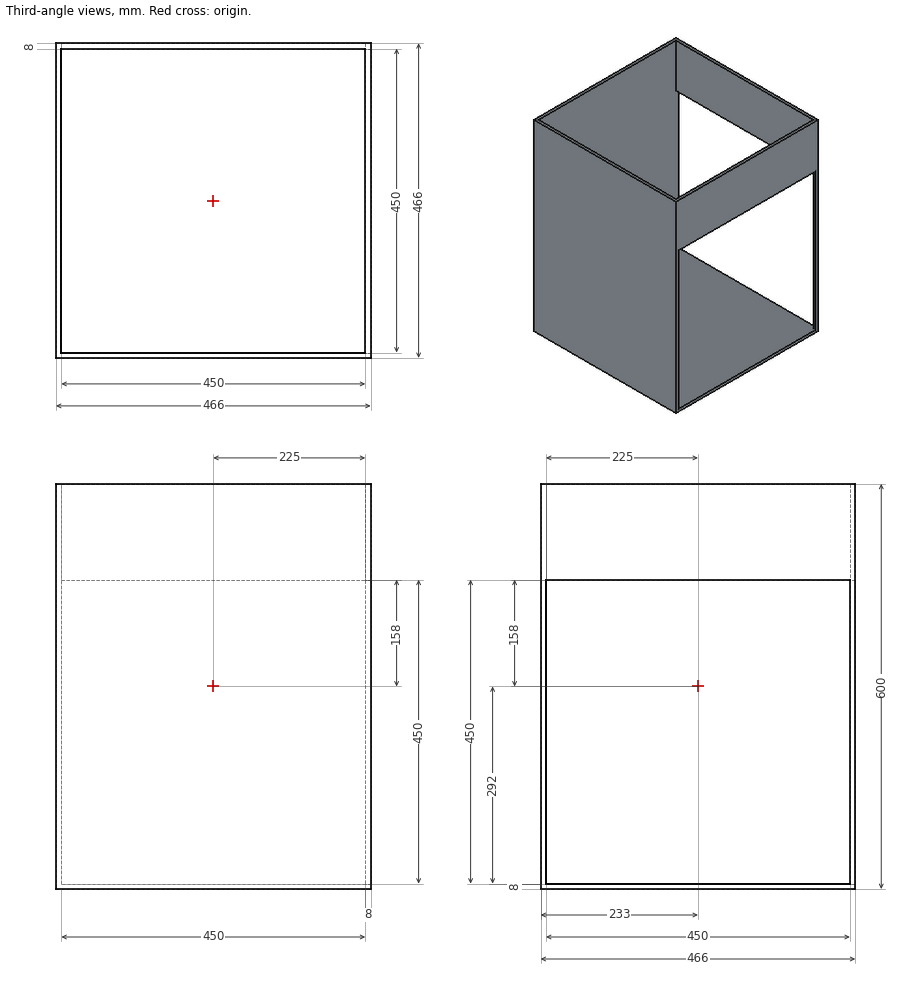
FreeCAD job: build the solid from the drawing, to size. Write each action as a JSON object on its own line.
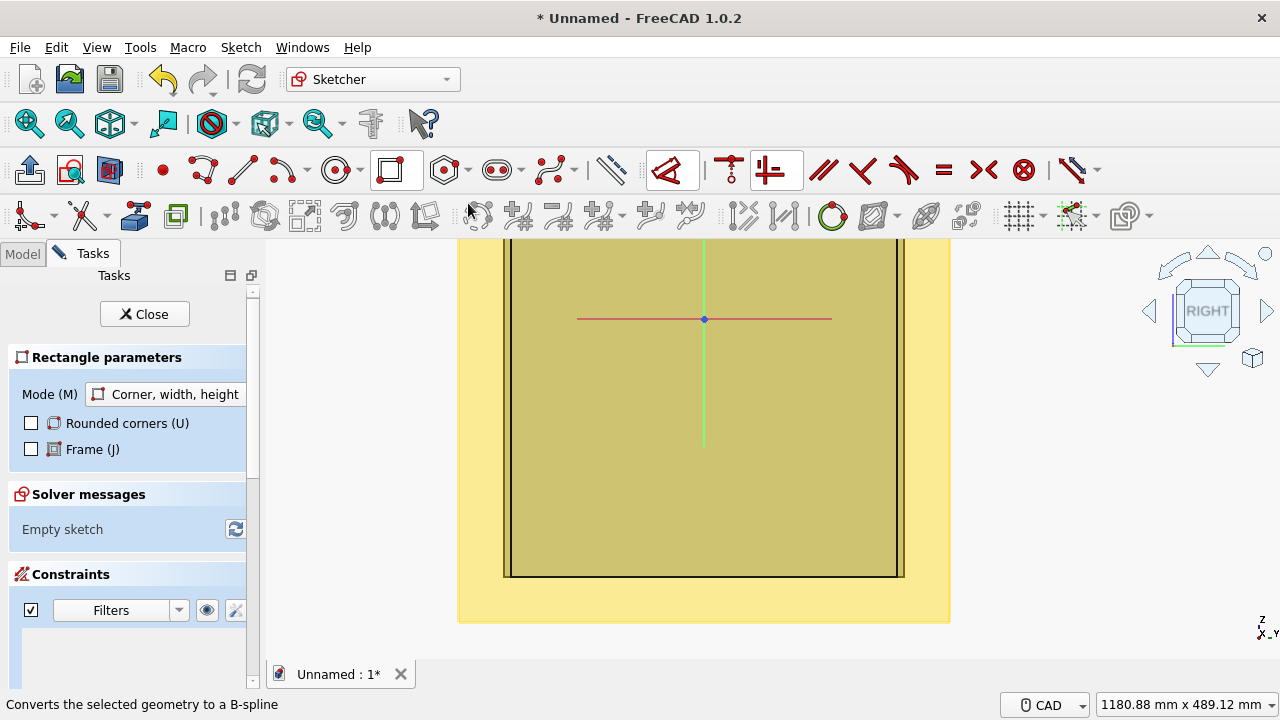
{"action": "scroll", "coordinate": [504, 570], "scroll_direction": "up", "scroll_amount": 5}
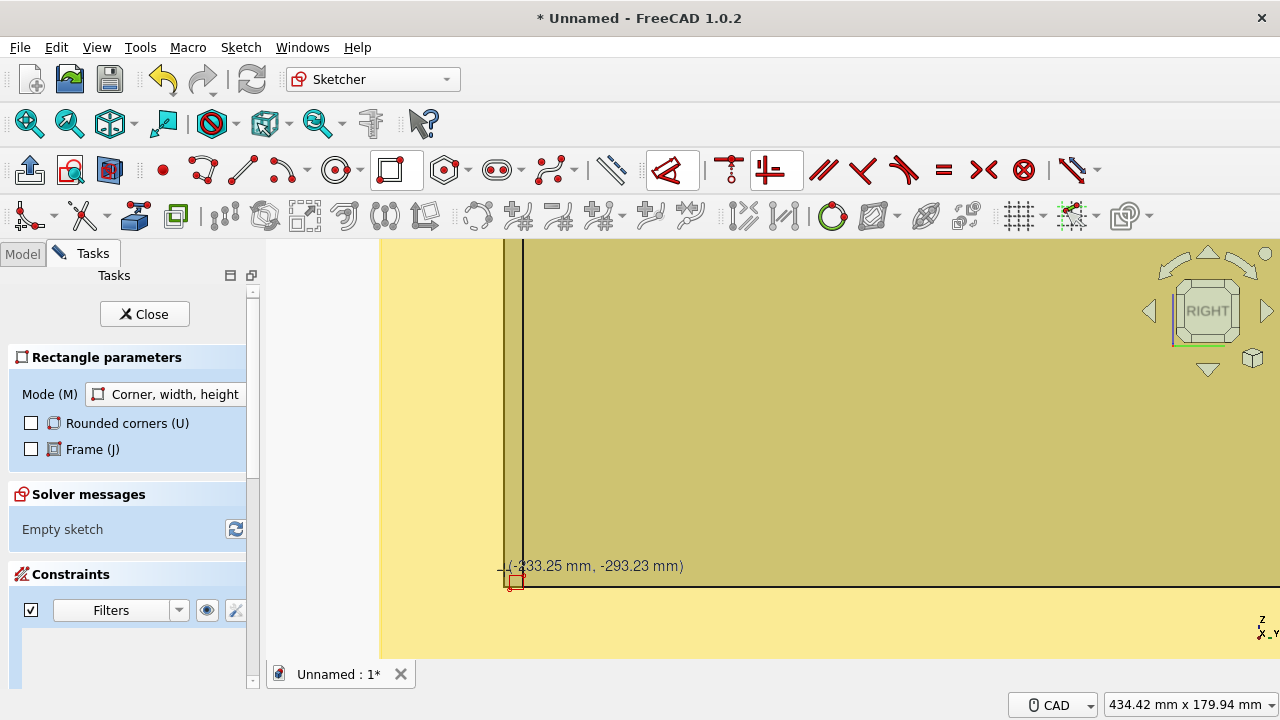
{"action": "left_click", "coordinate": [504, 568]}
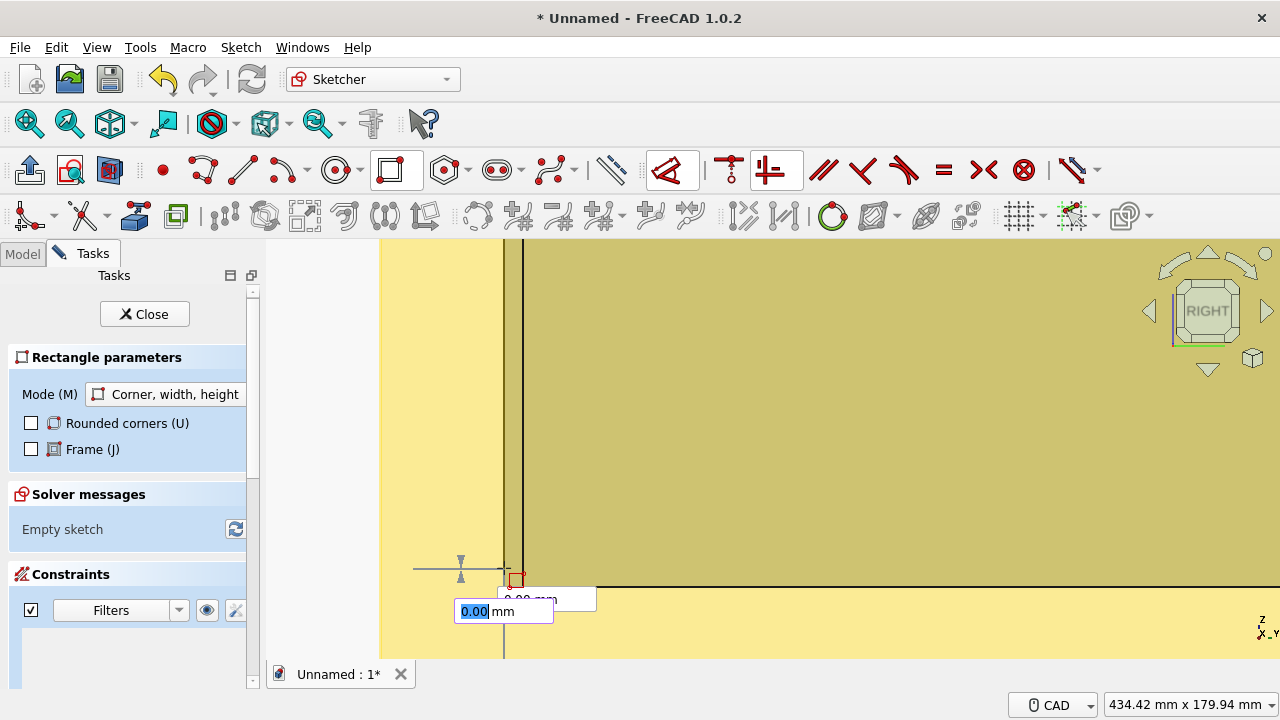
{"action": "scroll", "coordinate": [505, 572], "scroll_direction": "down", "scroll_amount": 5}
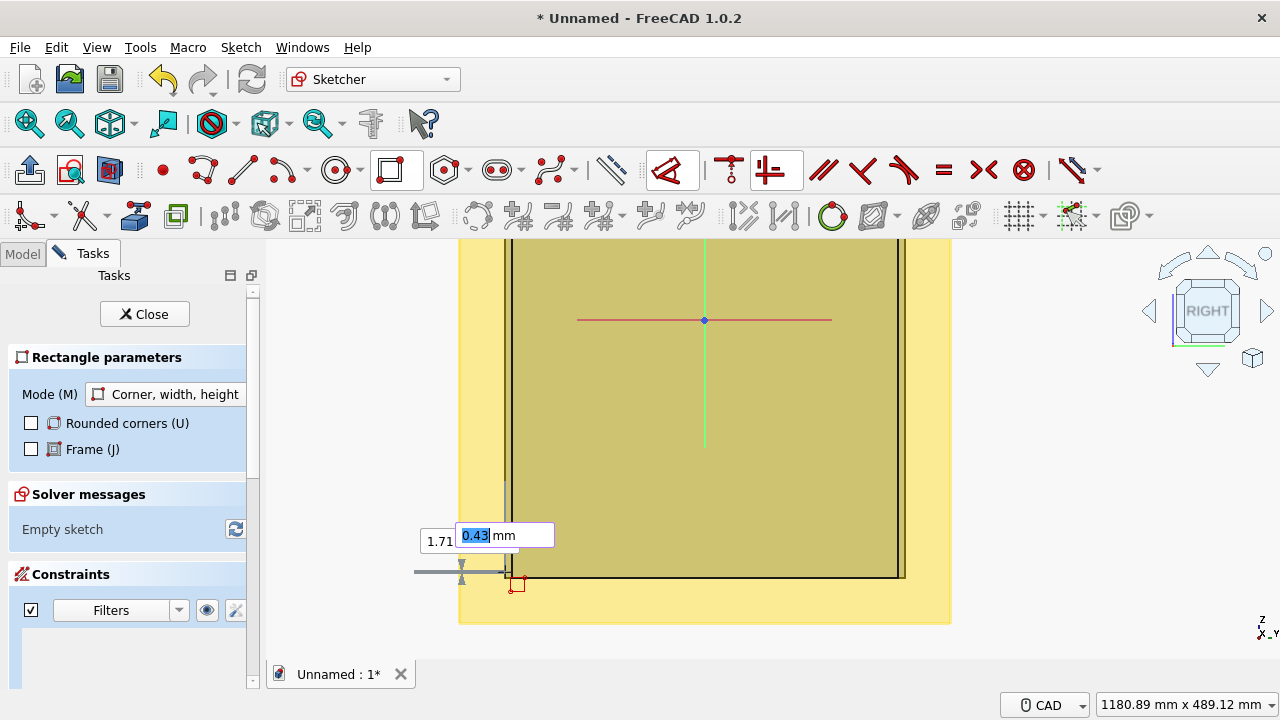
{"action": "left_click", "coordinate": [905, 578]}
{"action": "key", "text": "Escape"}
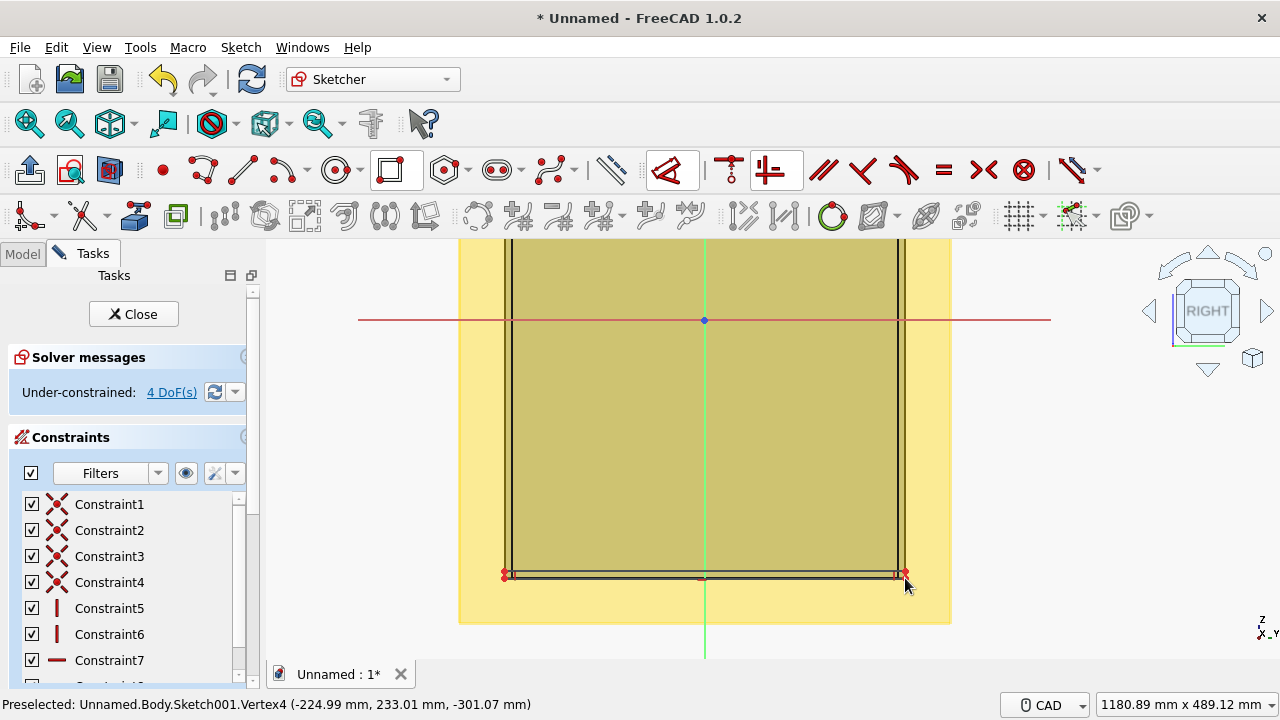
{"action": "scroll", "coordinate": [505, 575], "scroll_direction": "up", "scroll_amount": 9}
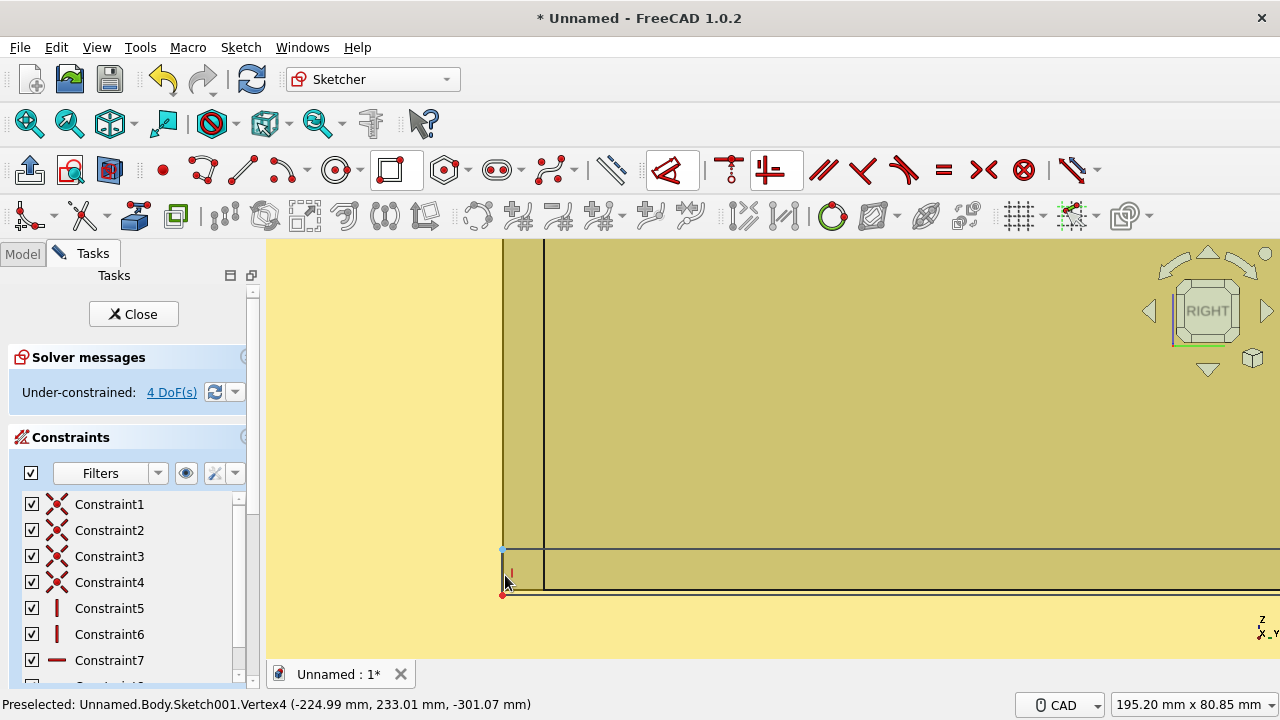
{"action": "left_click", "coordinate": [502, 572]}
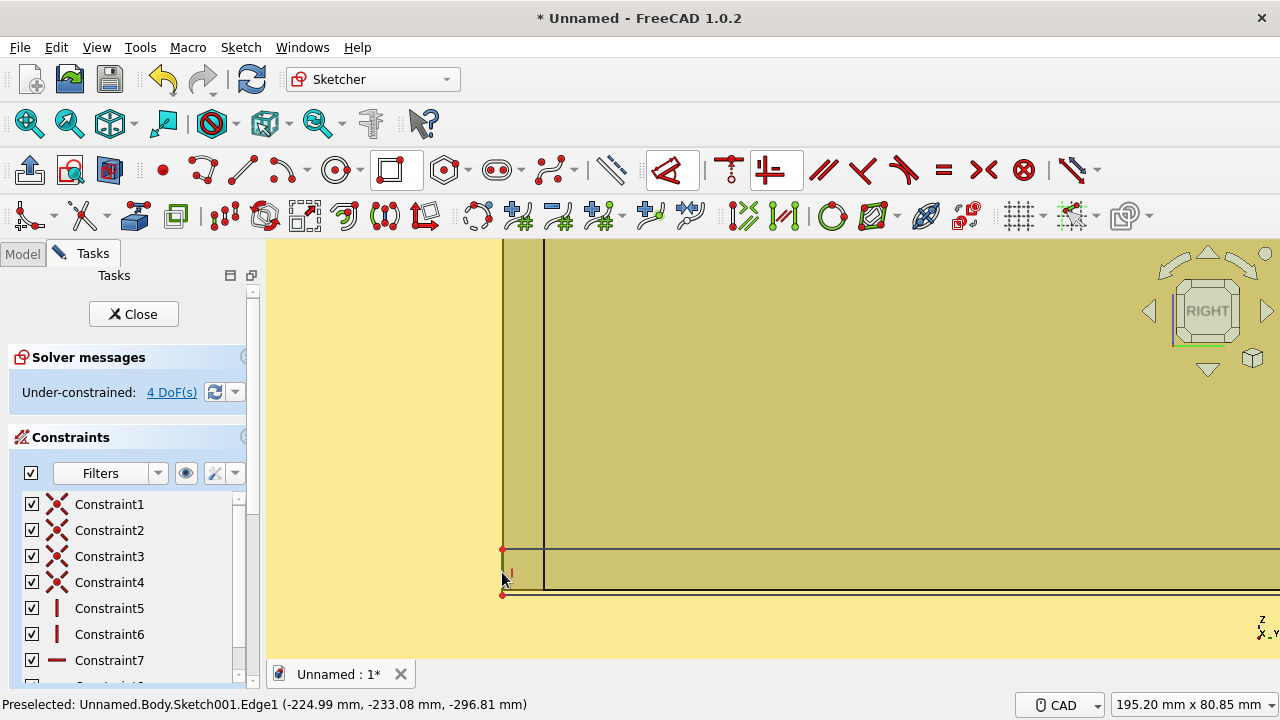
{"action": "key", "text": "i"}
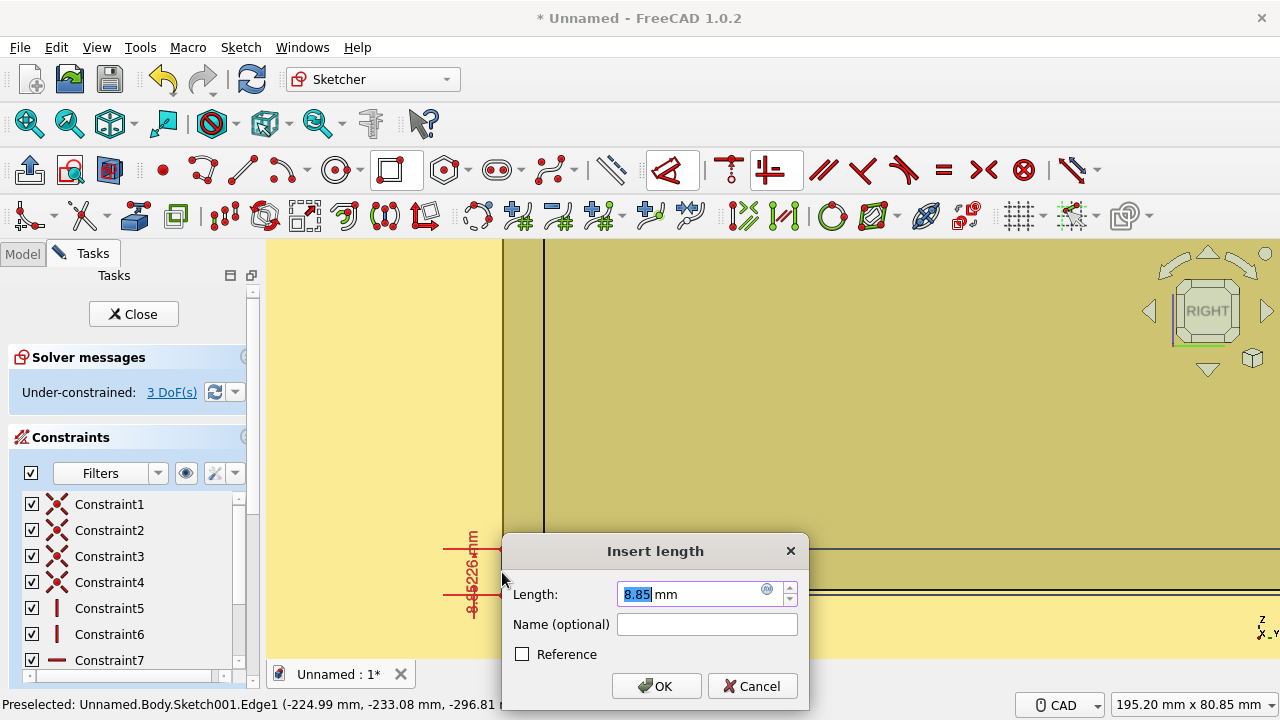
{"action": "type", "text": "8"}
{"action": "key", "text": "Return"}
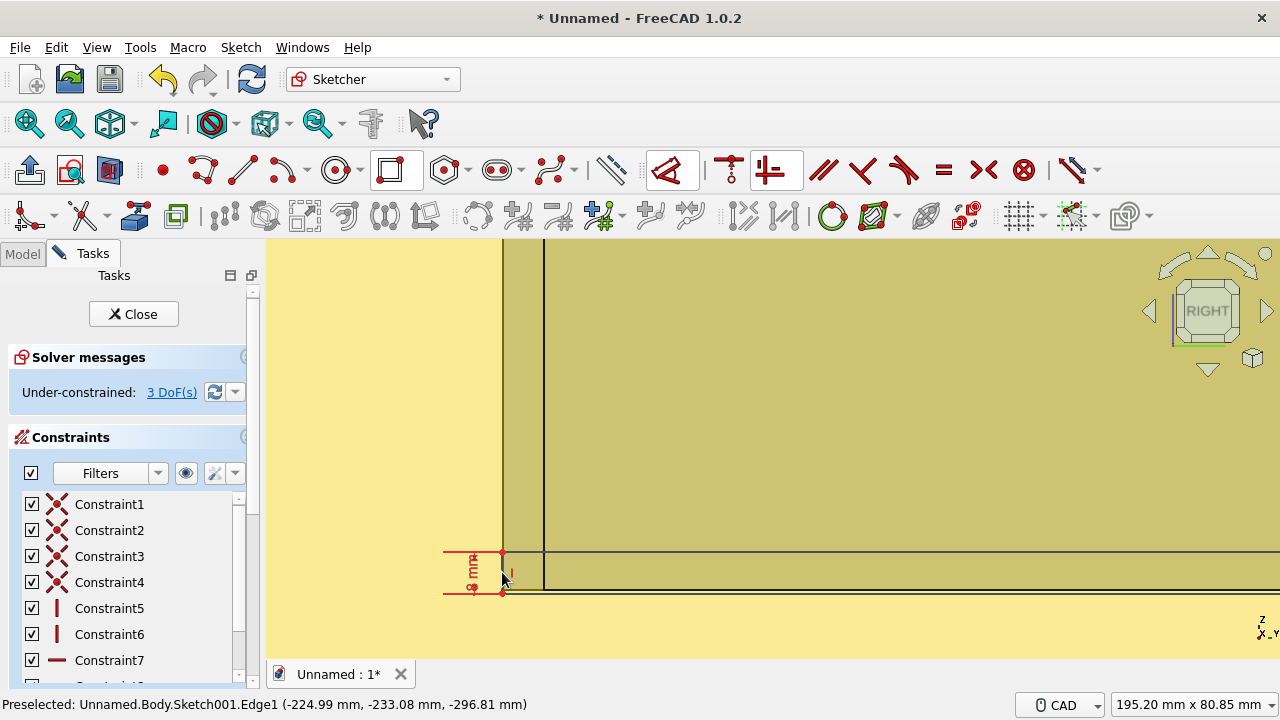
{"action": "scroll", "coordinate": [505, 575], "scroll_direction": "down", "scroll_amount": 9}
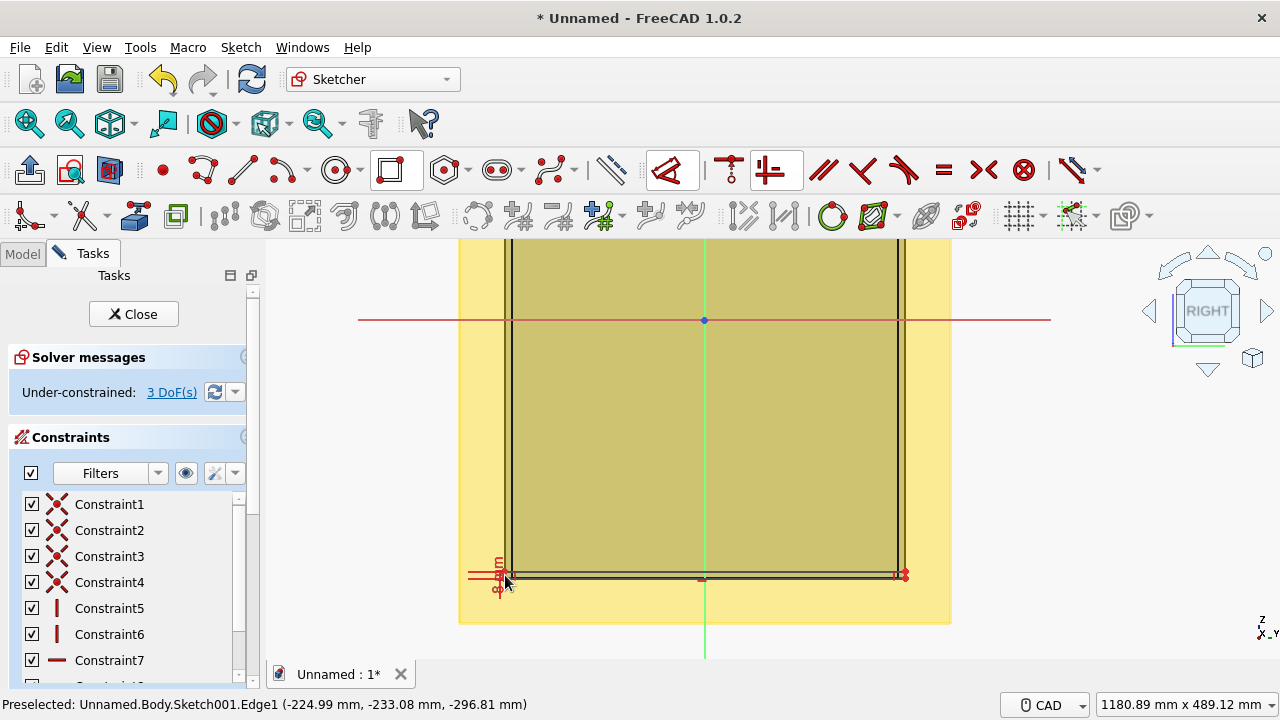
{"action": "scroll", "coordinate": [585, 579], "scroll_direction": "up", "scroll_amount": 4}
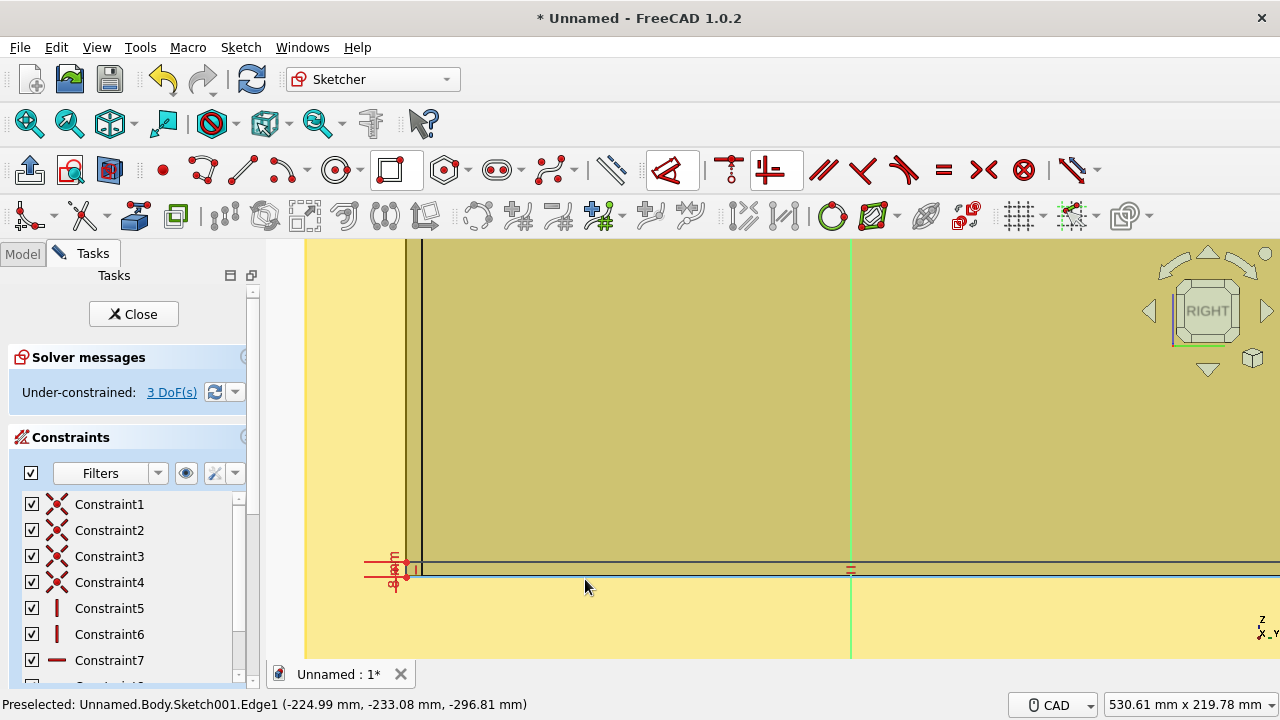
{"action": "left_click", "coordinate": [584, 577]}